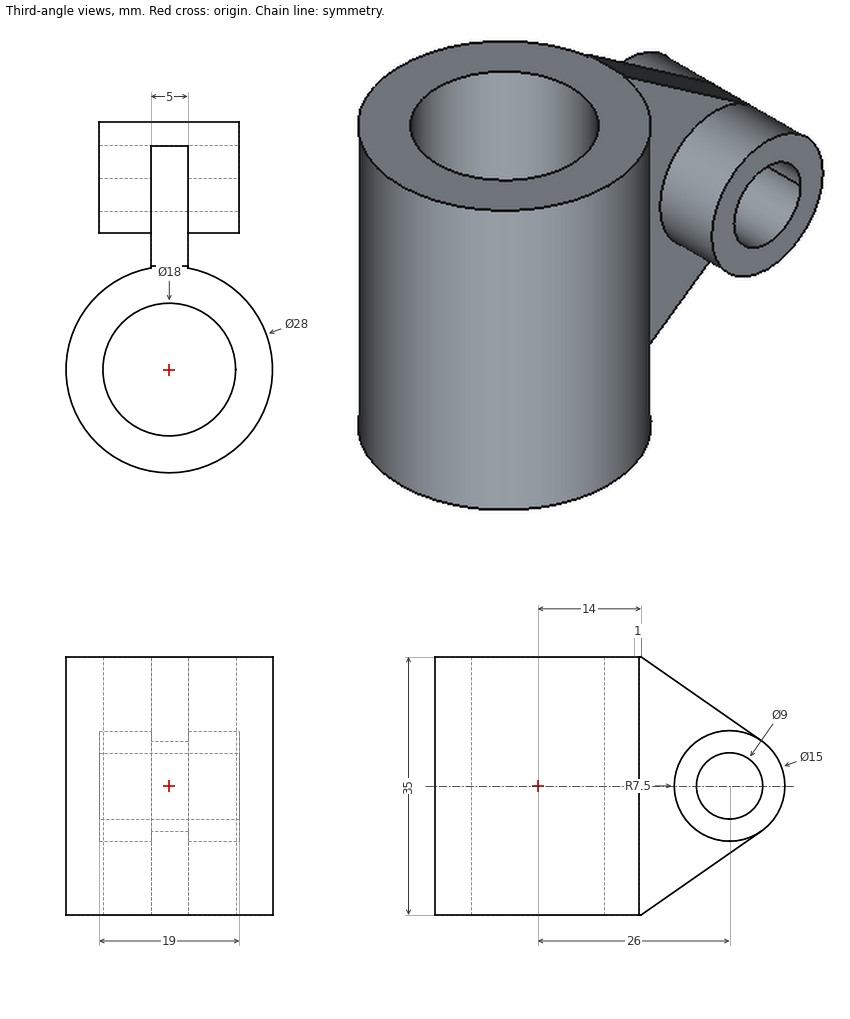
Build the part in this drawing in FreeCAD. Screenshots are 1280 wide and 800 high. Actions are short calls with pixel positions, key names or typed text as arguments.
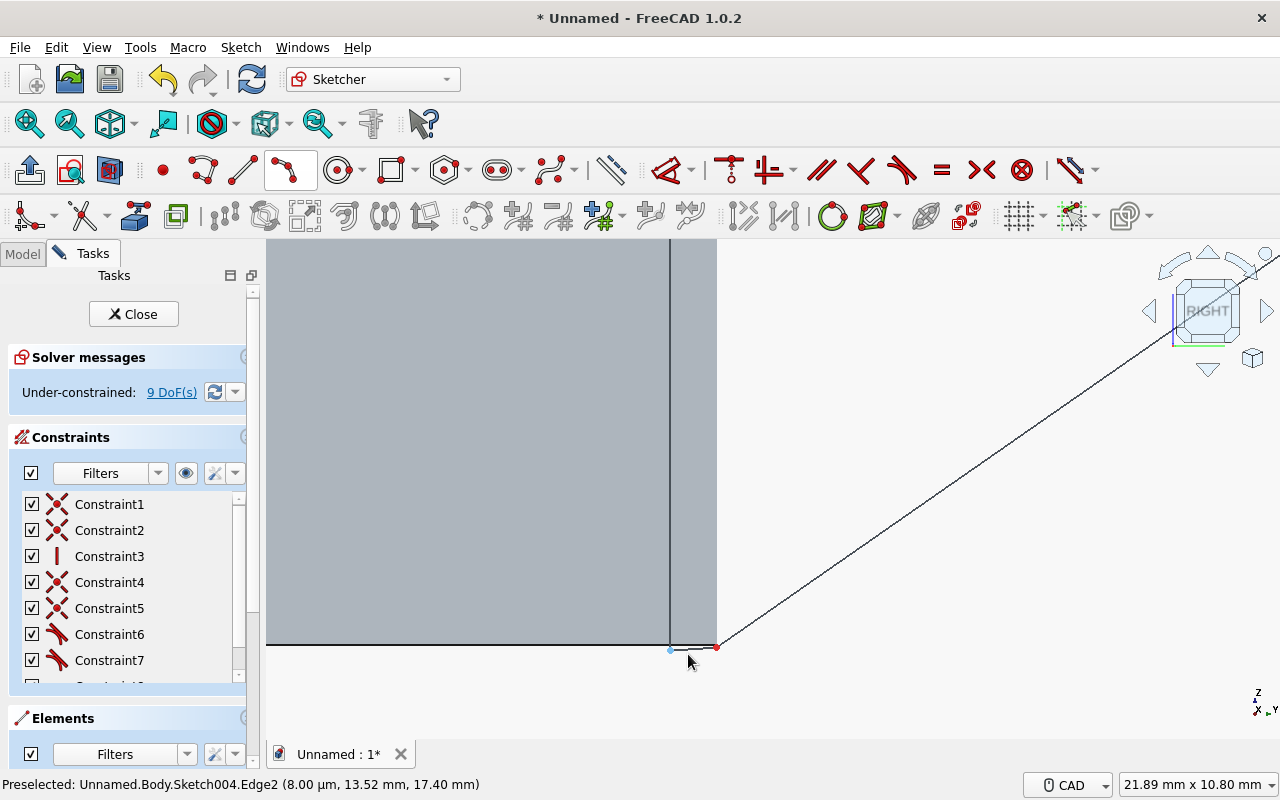
click(684, 650)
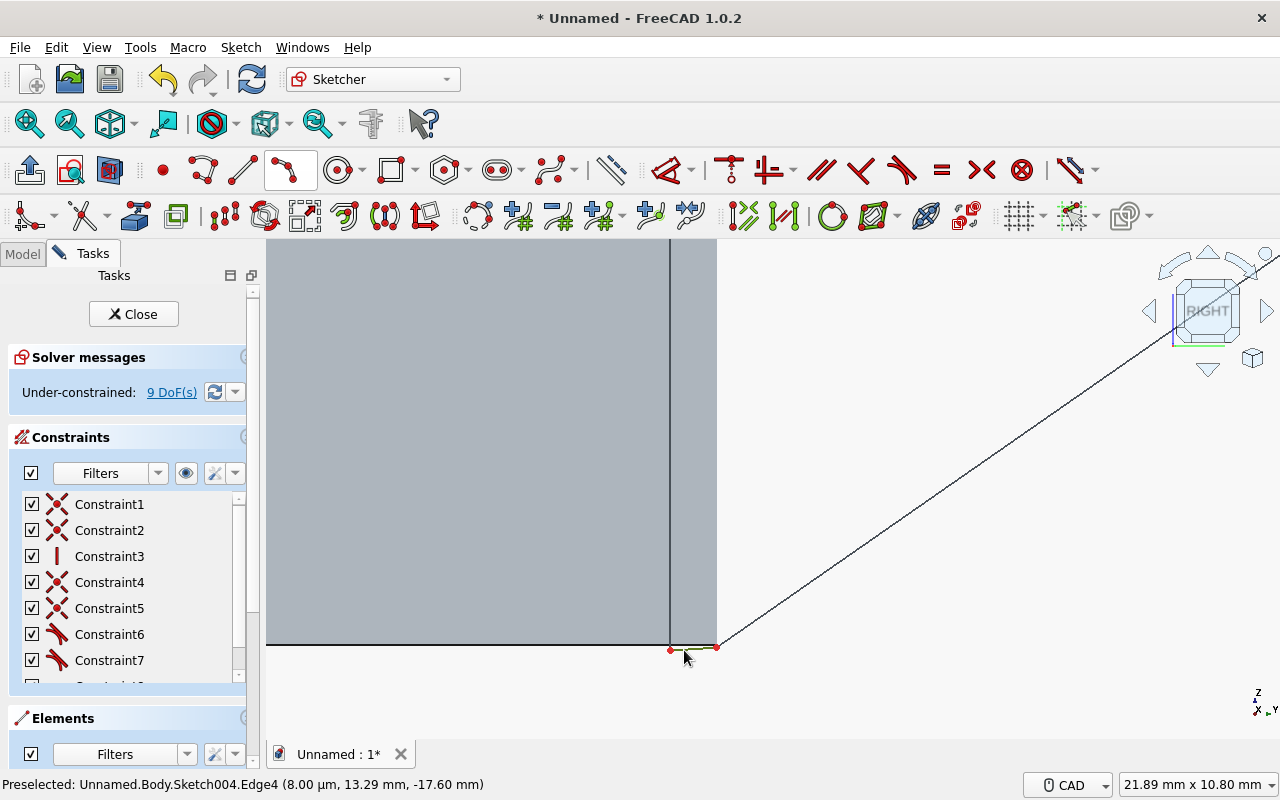
key(h)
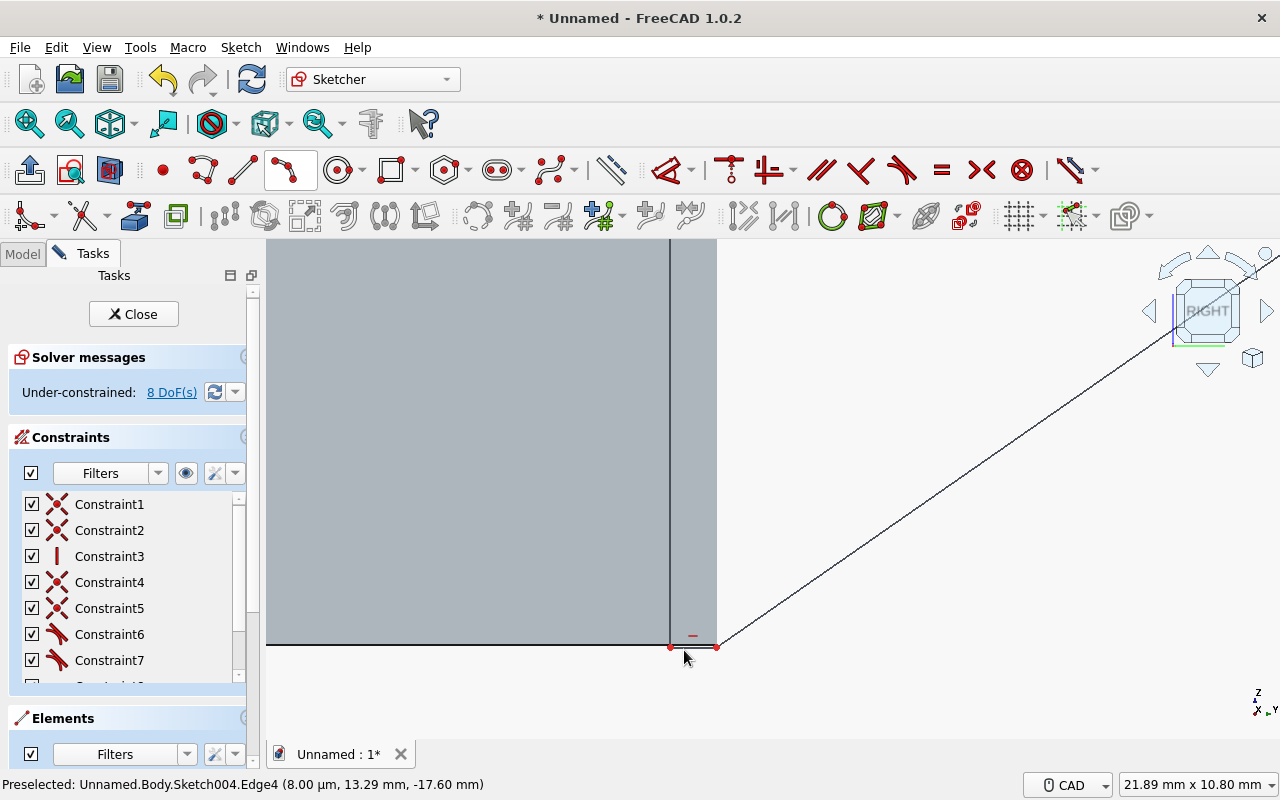
scroll(688, 655, down, 8)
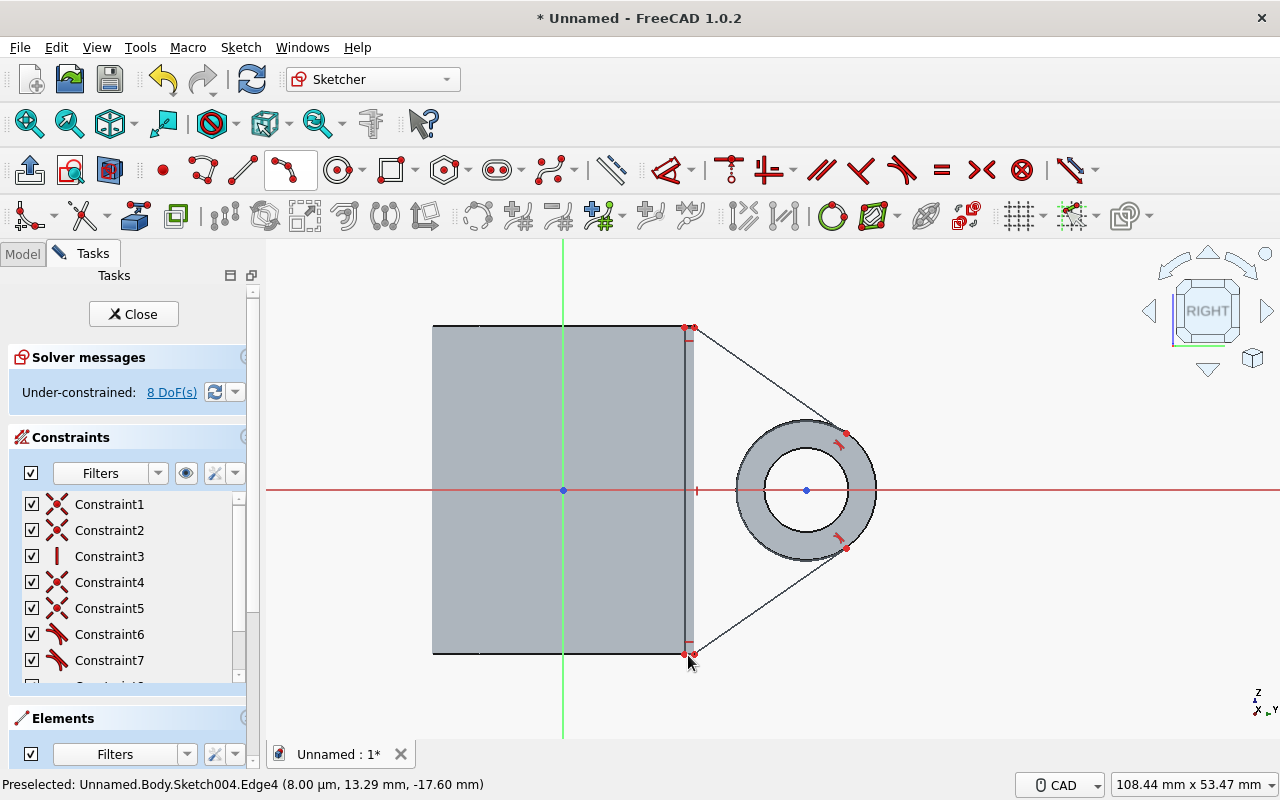
click(806, 491)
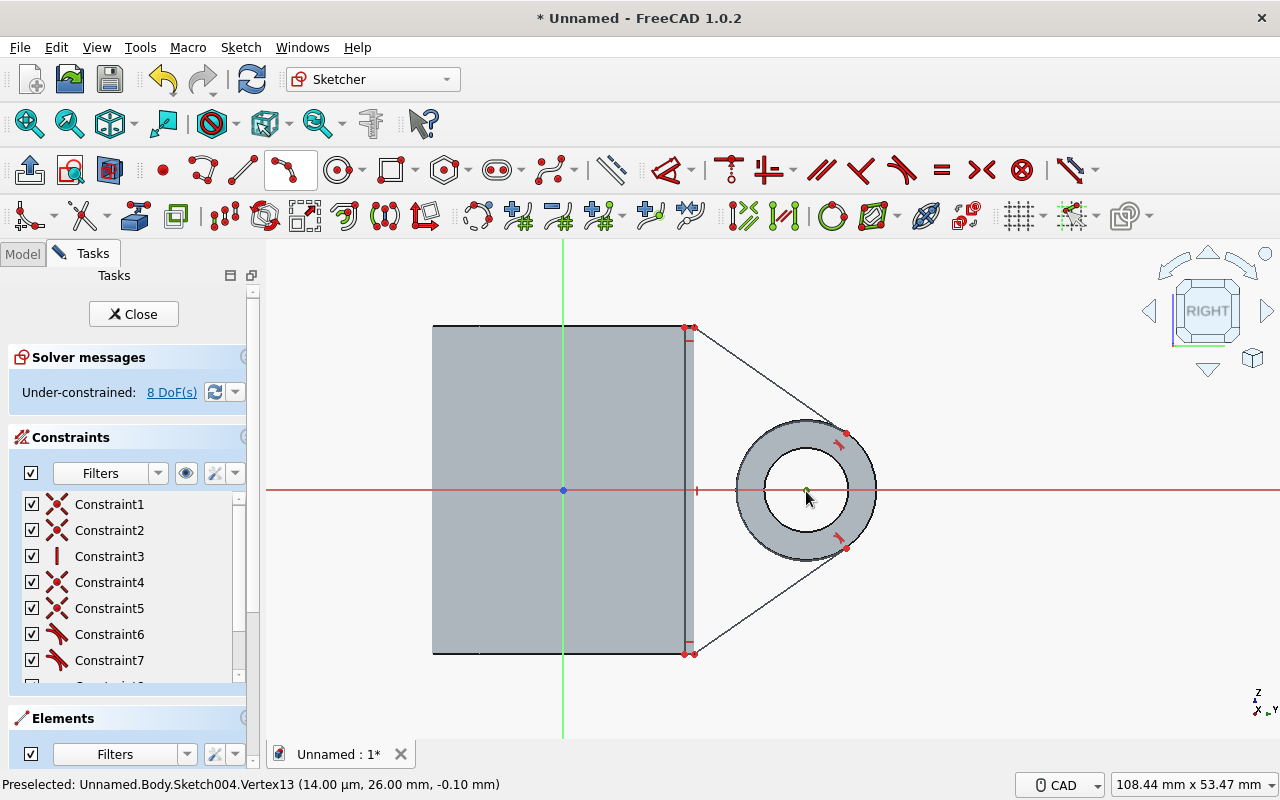
click(353, 490)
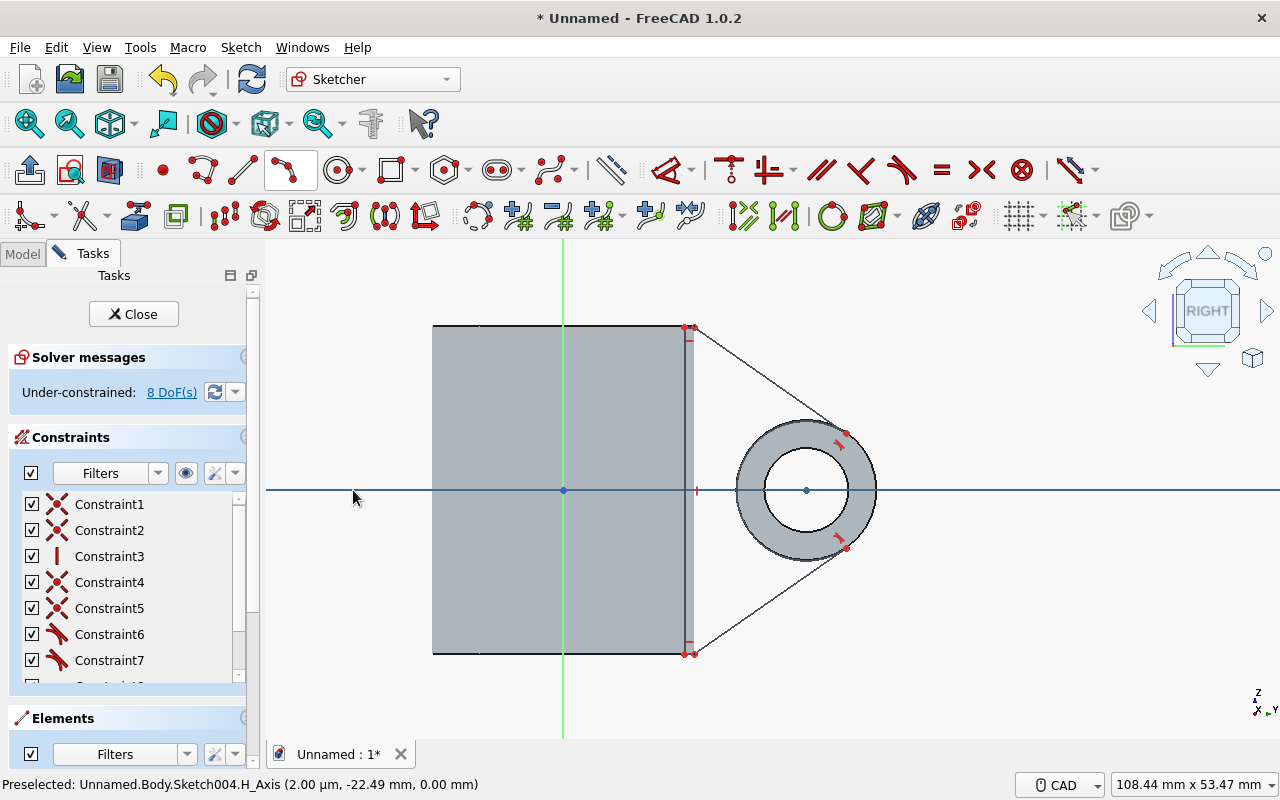
key(c)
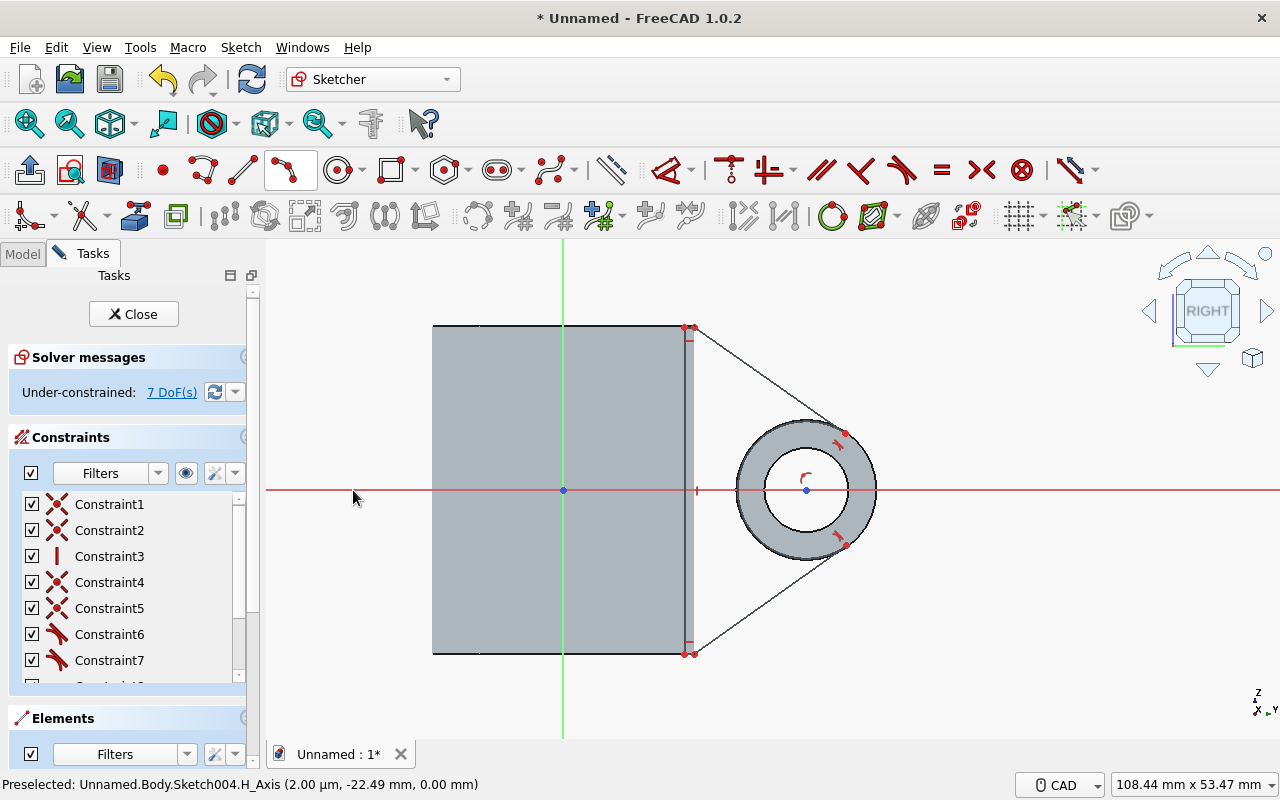
scroll(695, 328, up, 2)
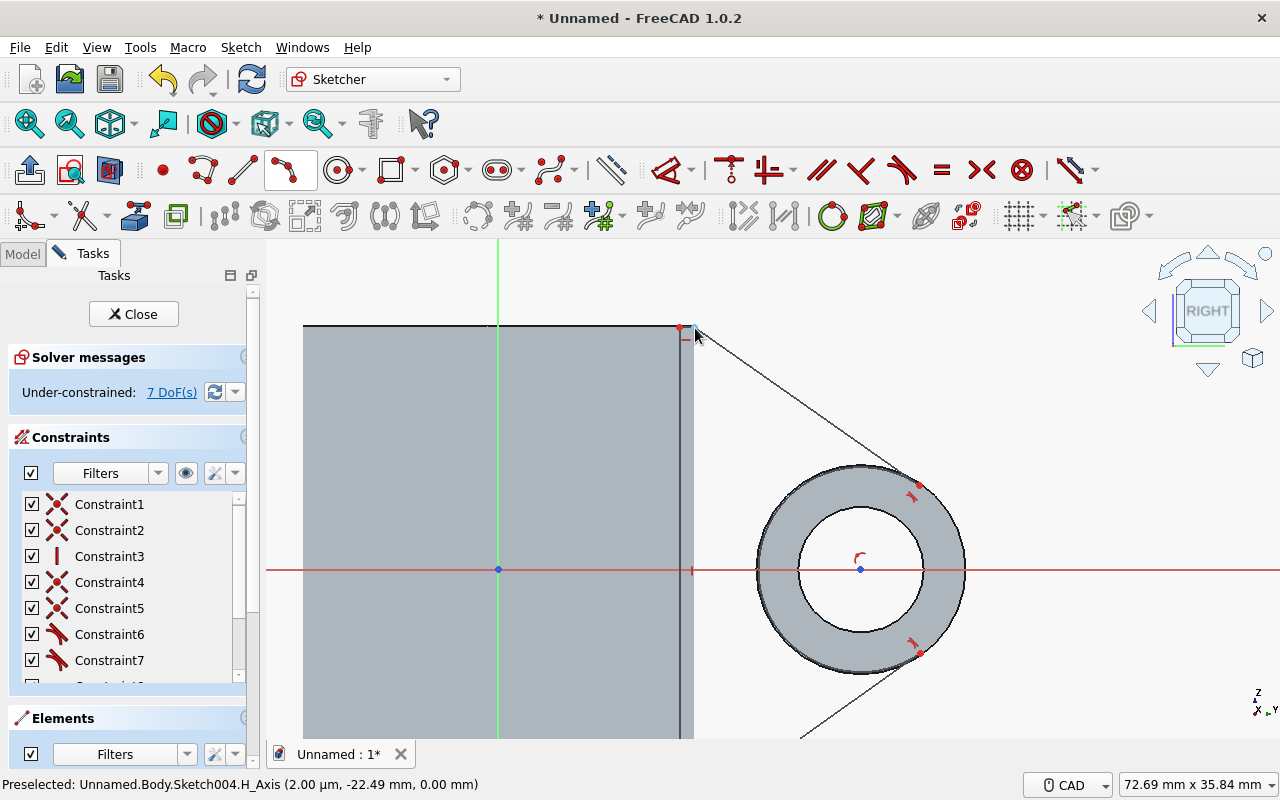
click(694, 327)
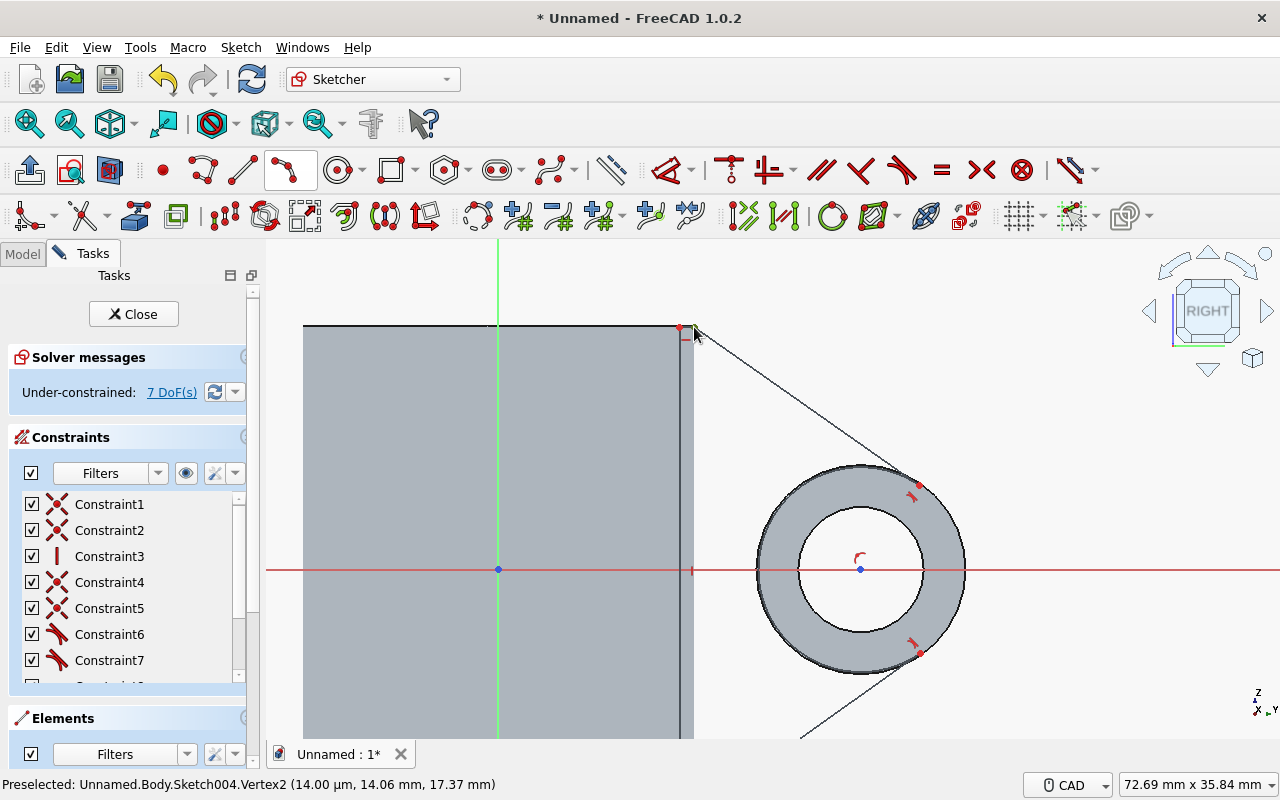
scroll(694, 325, down, 2)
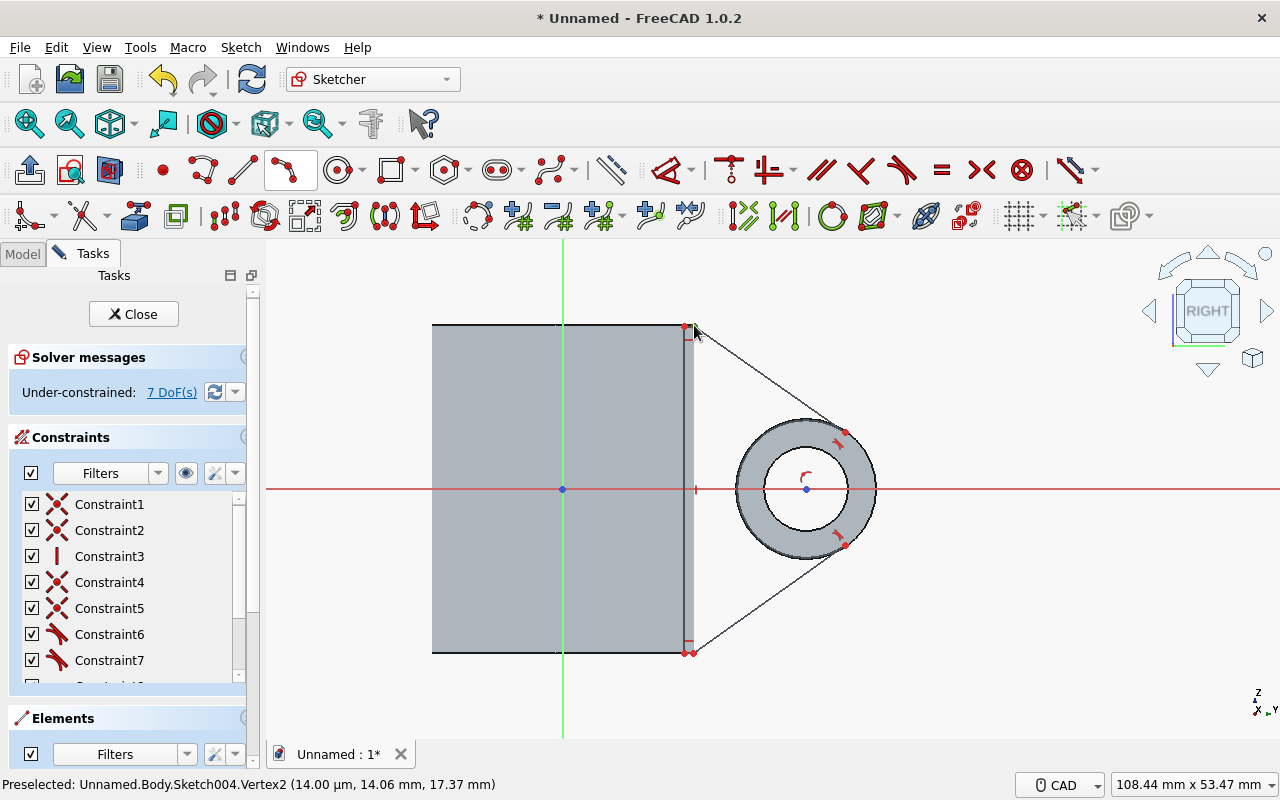
scroll(694, 653, up, 2)